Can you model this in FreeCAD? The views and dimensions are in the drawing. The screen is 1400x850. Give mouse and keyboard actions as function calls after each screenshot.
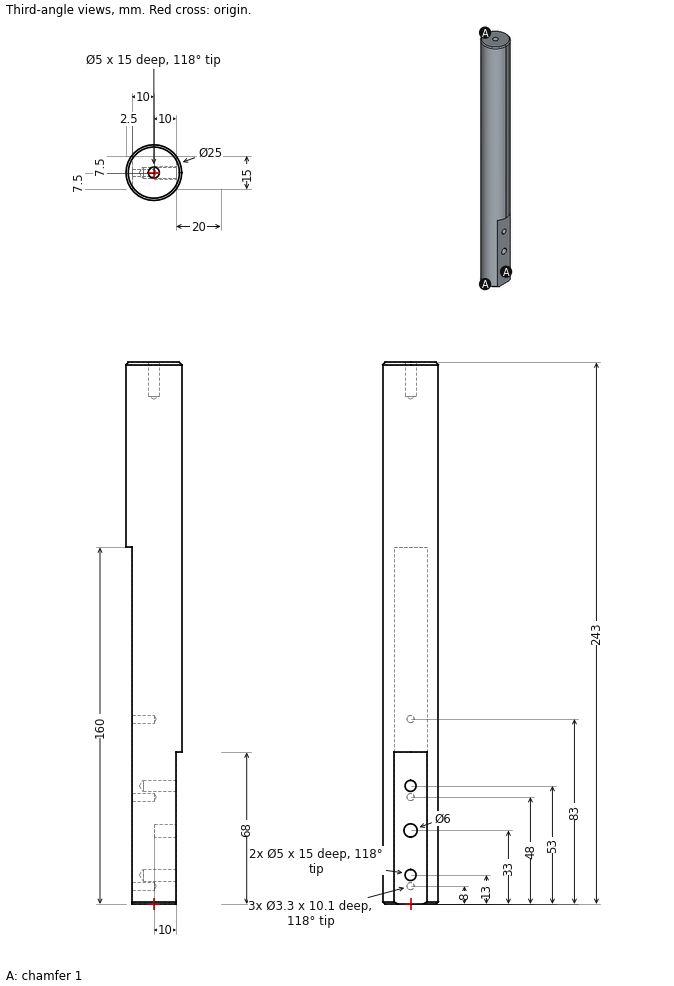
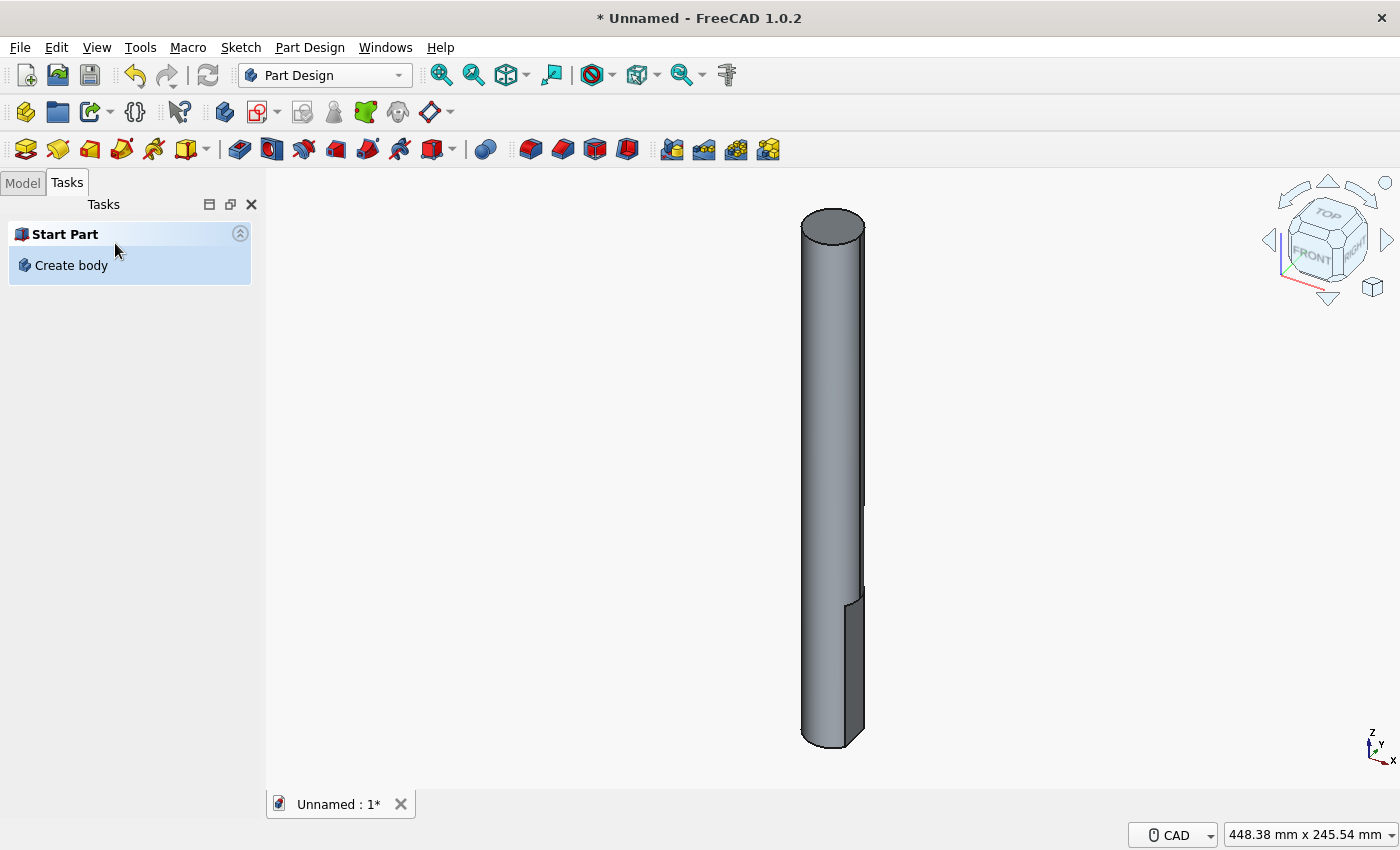
click(833, 226)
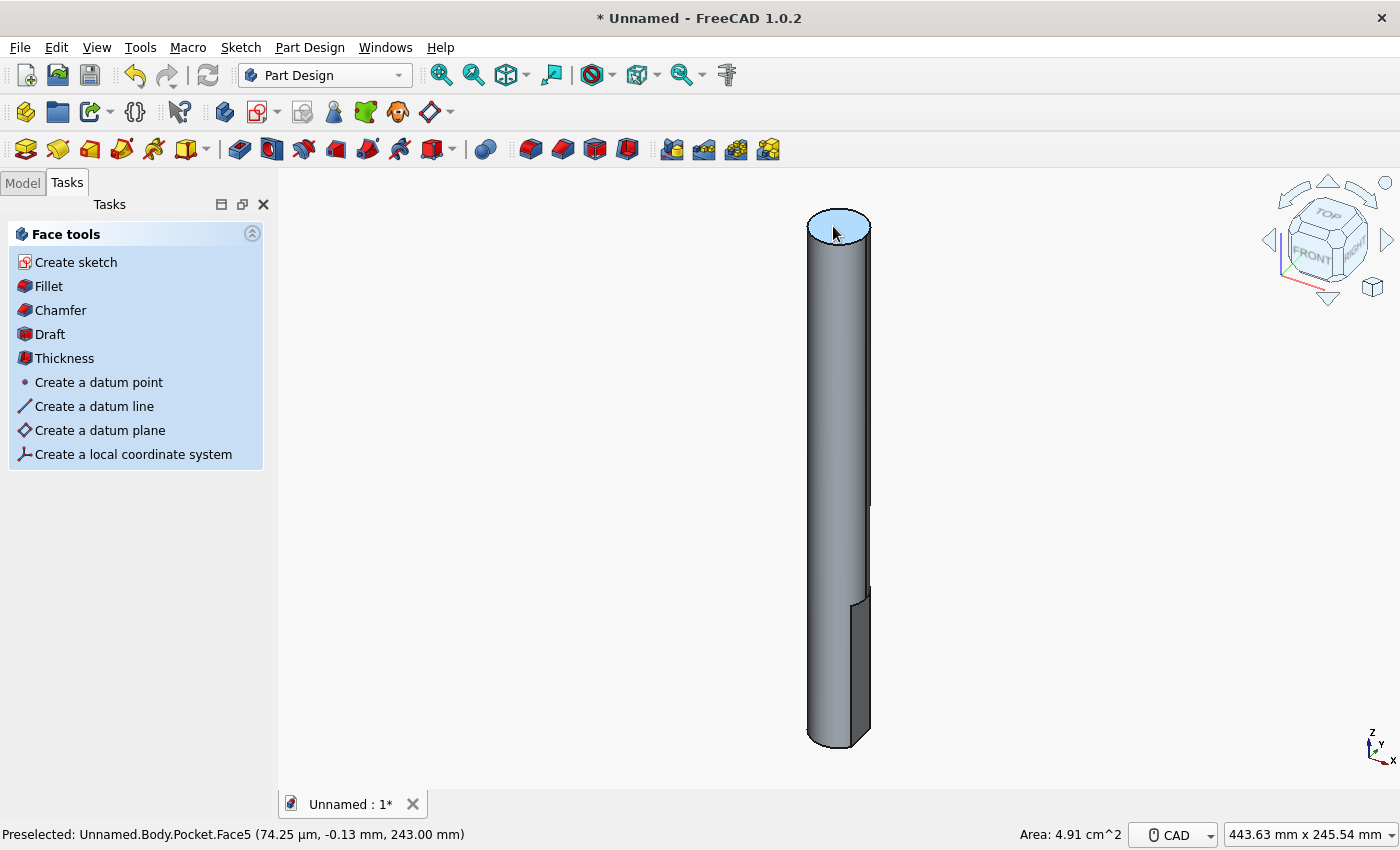
click(258, 112)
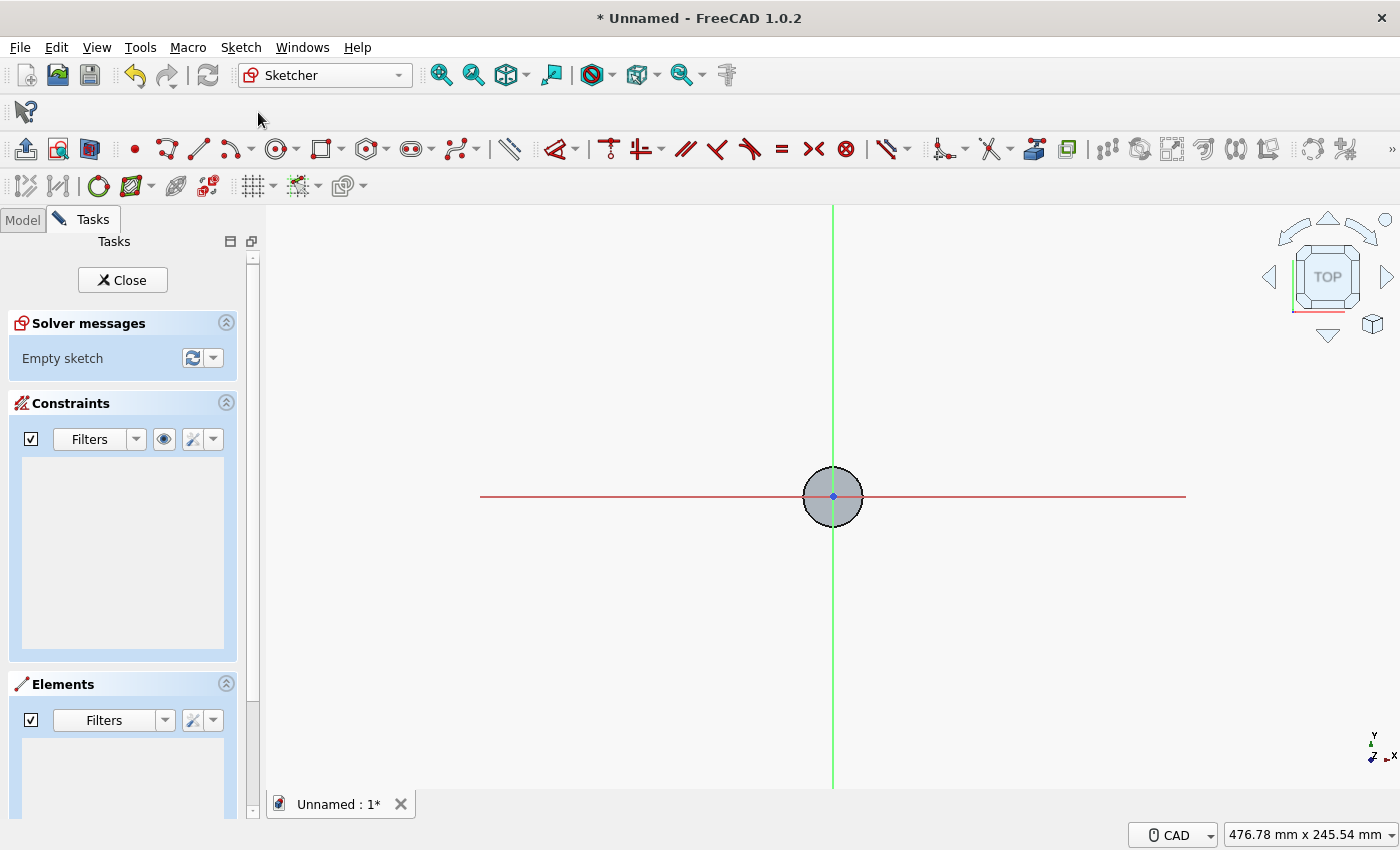
scroll(837, 497, up, 15)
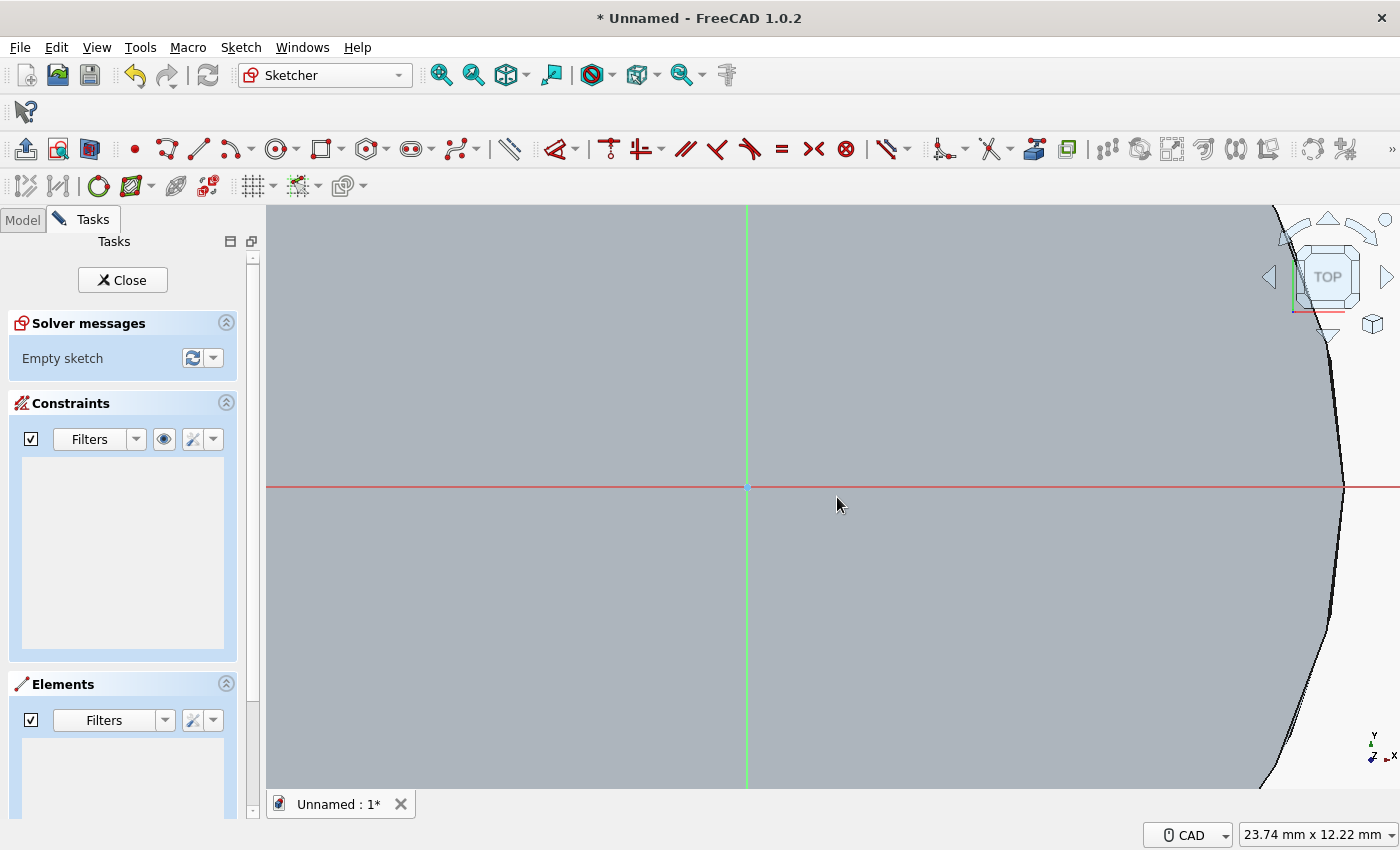
scroll(712, 468, up, 2)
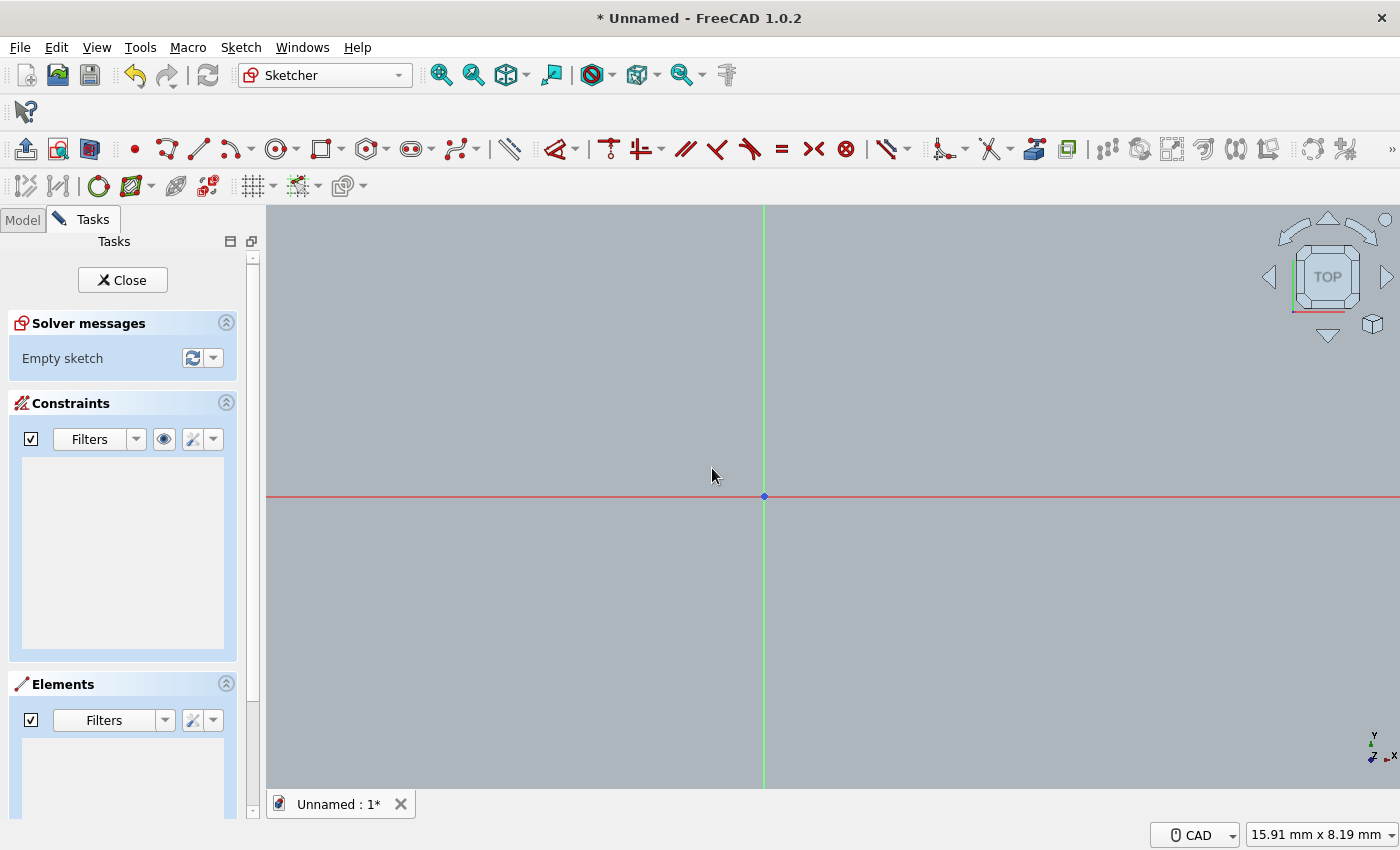
key(g)
key(c)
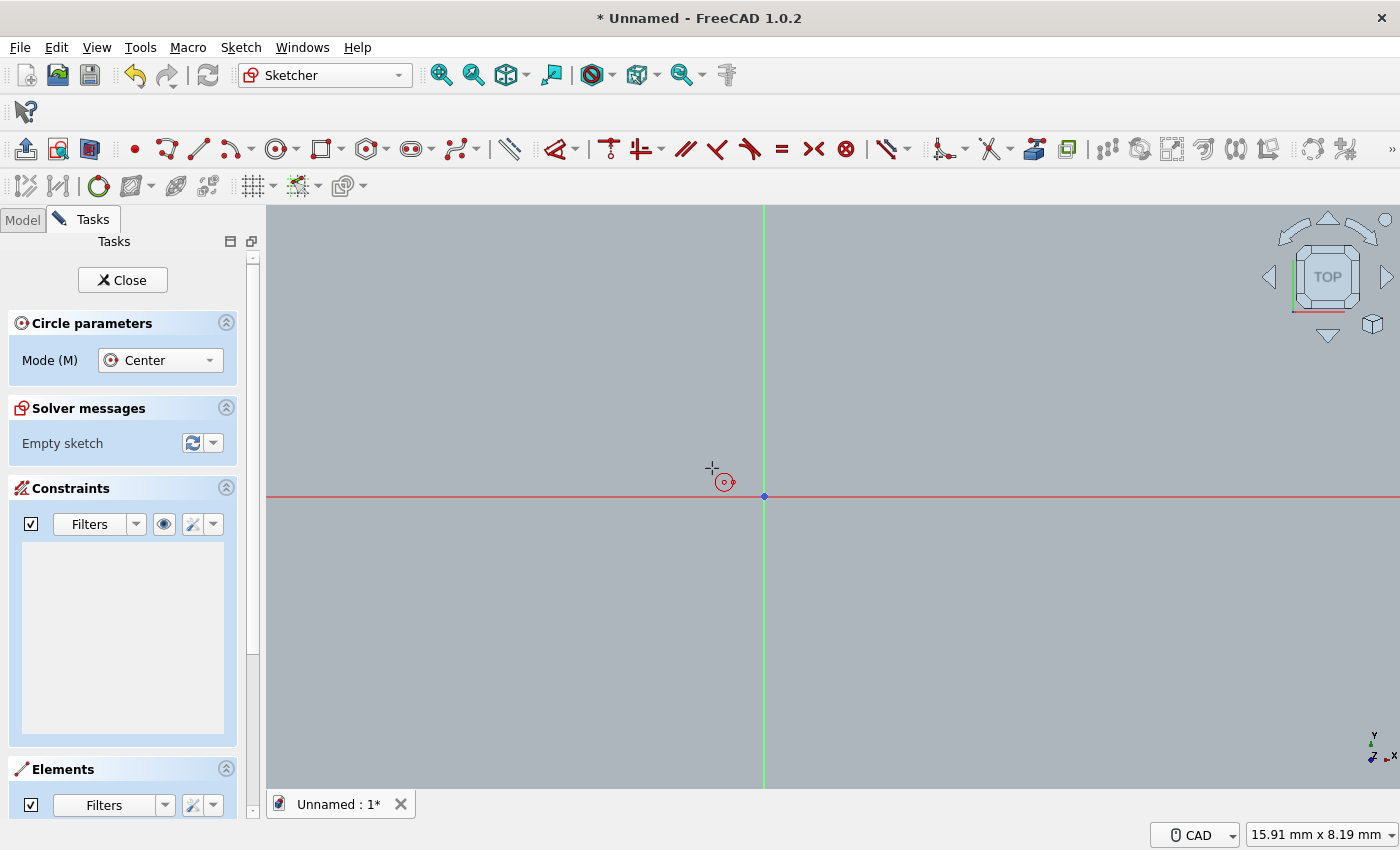
click(764, 497)
click(890, 371)
key(Escape)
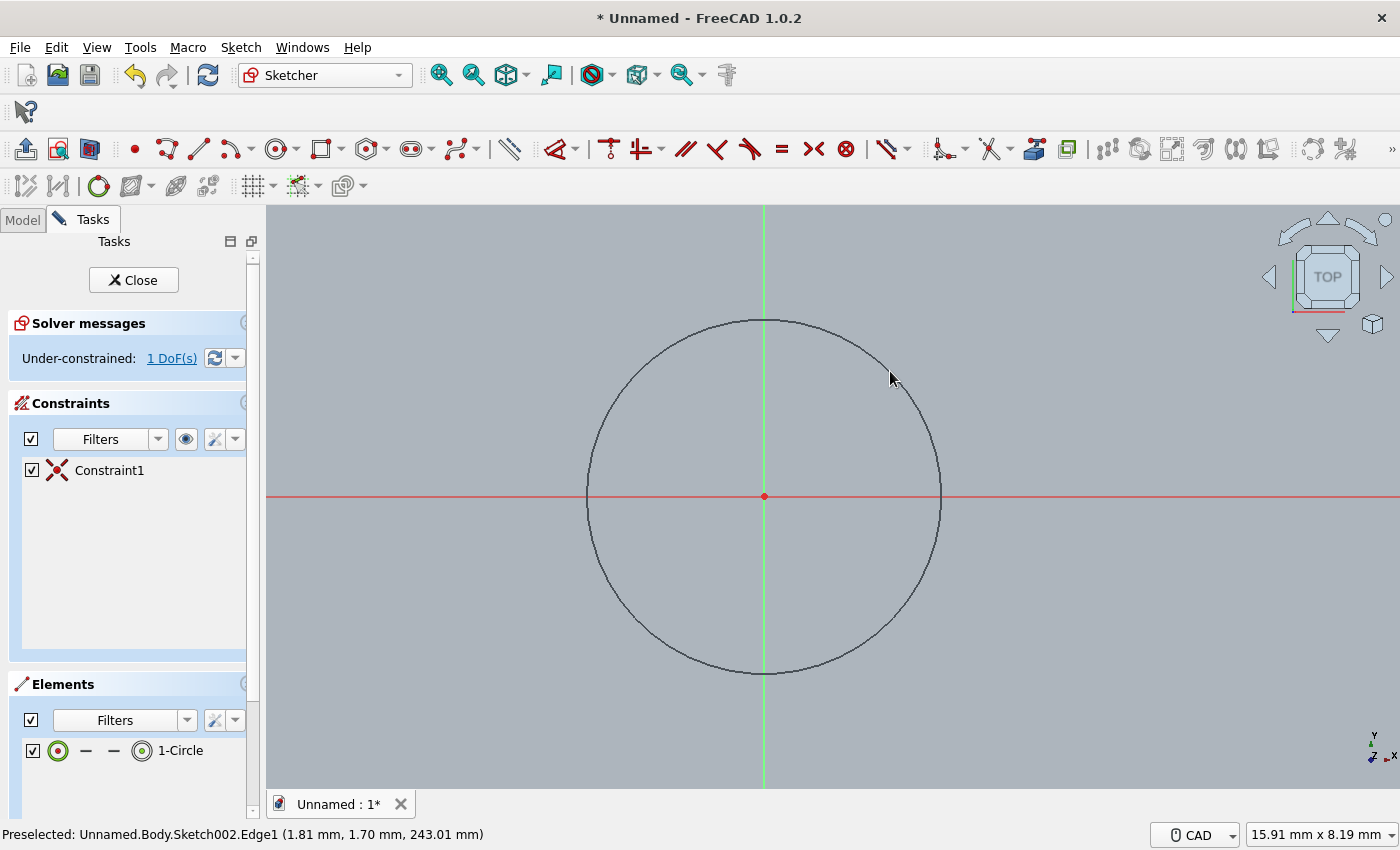
click(556, 150)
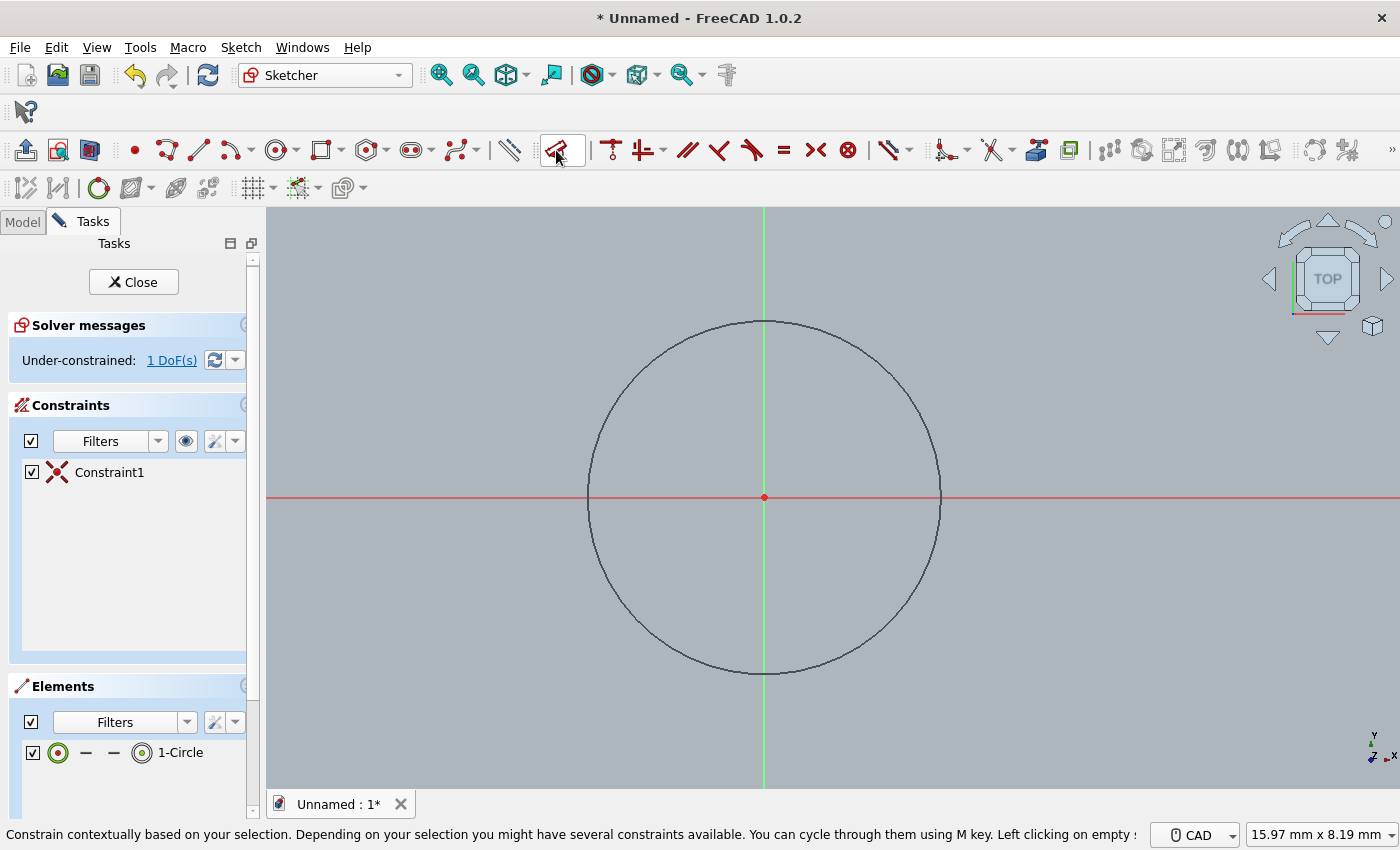
click(889, 372)
click(912, 349)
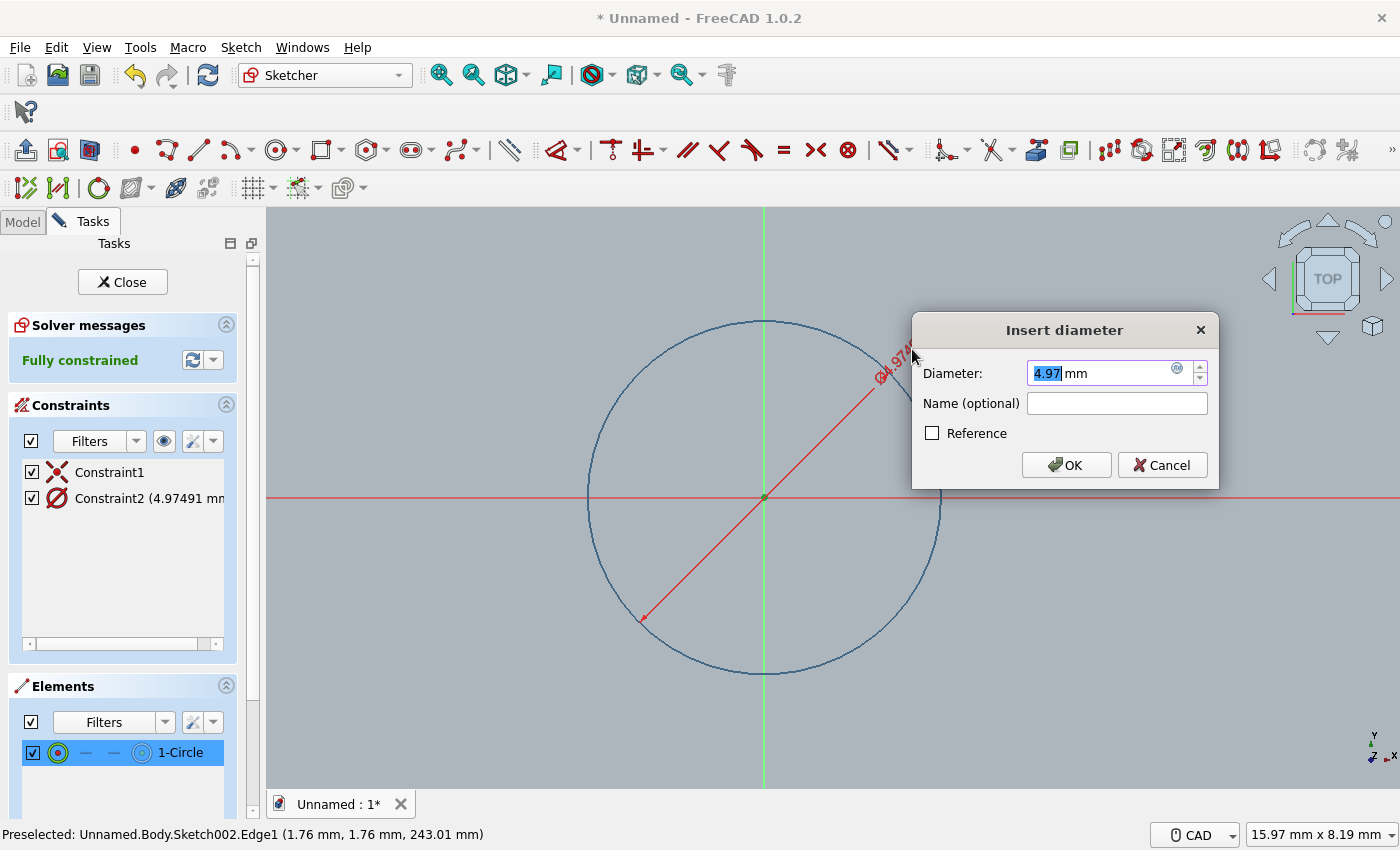
text(5)
key(Return)
key(Escape)